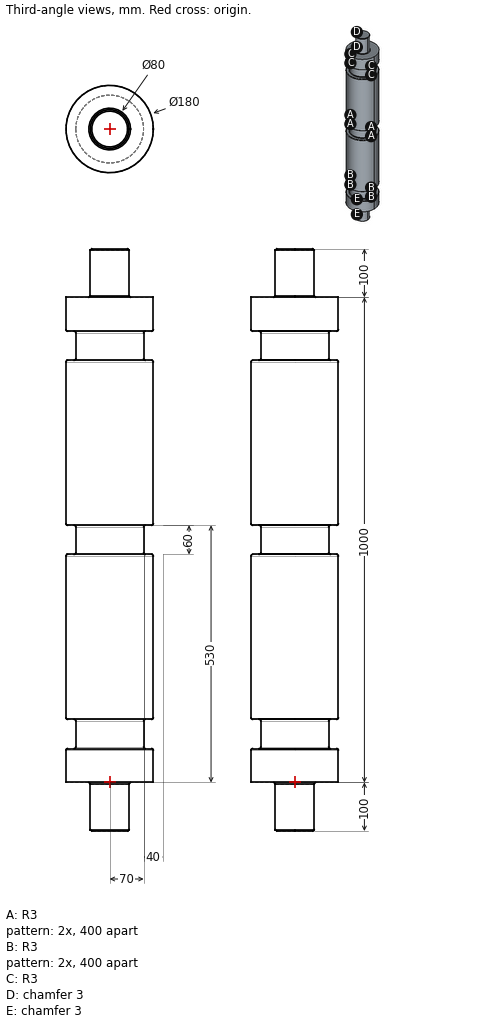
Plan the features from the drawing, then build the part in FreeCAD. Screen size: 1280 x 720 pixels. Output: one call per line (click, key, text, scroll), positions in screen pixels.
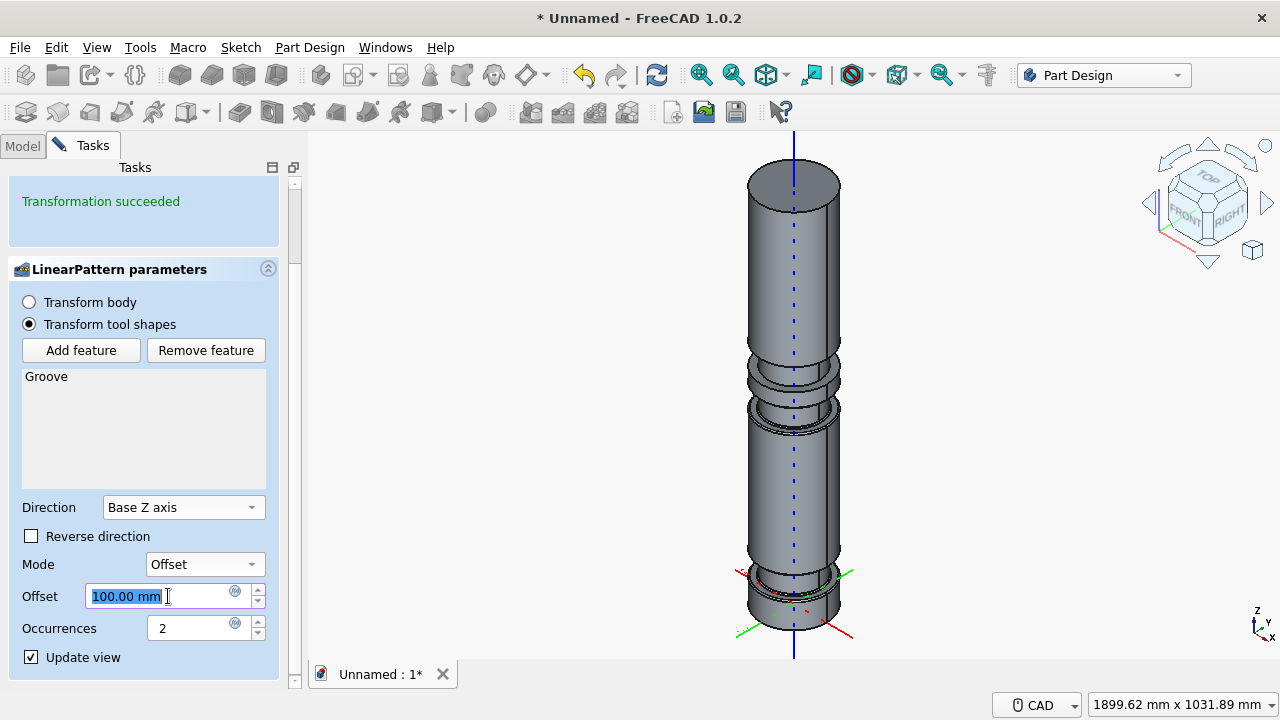
text(400)
key(Tab)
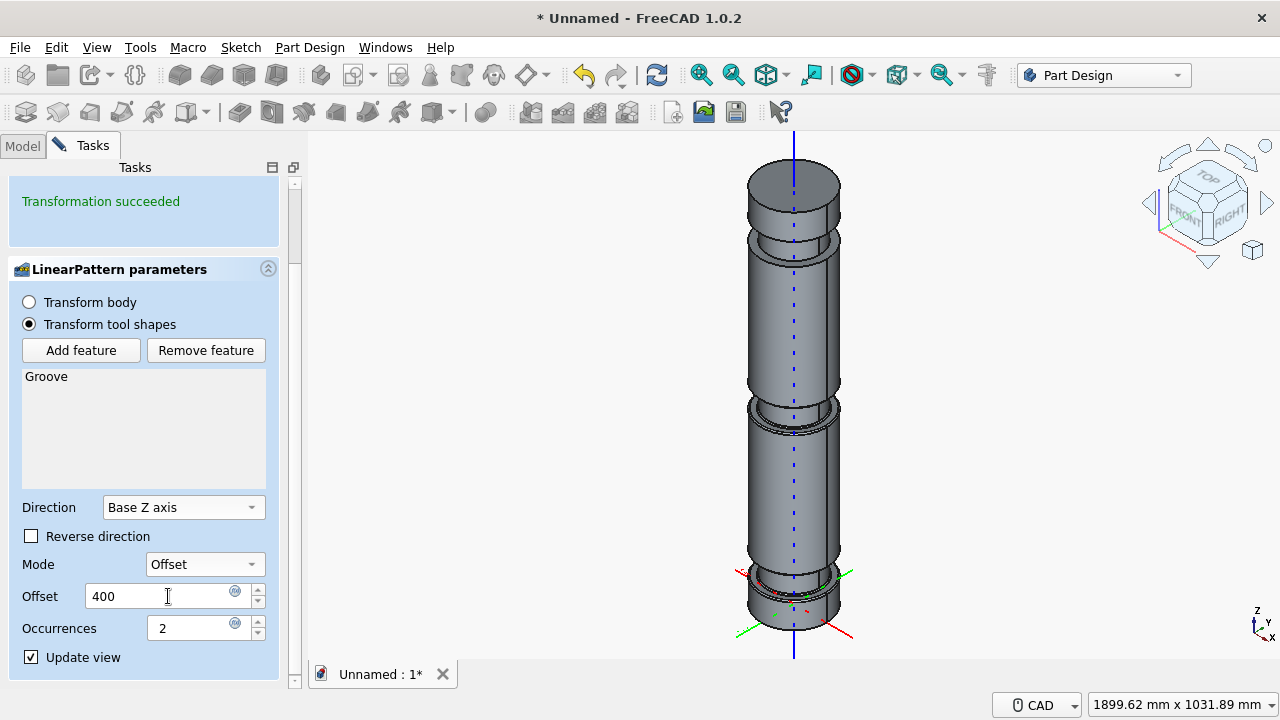
triple_click(198, 628)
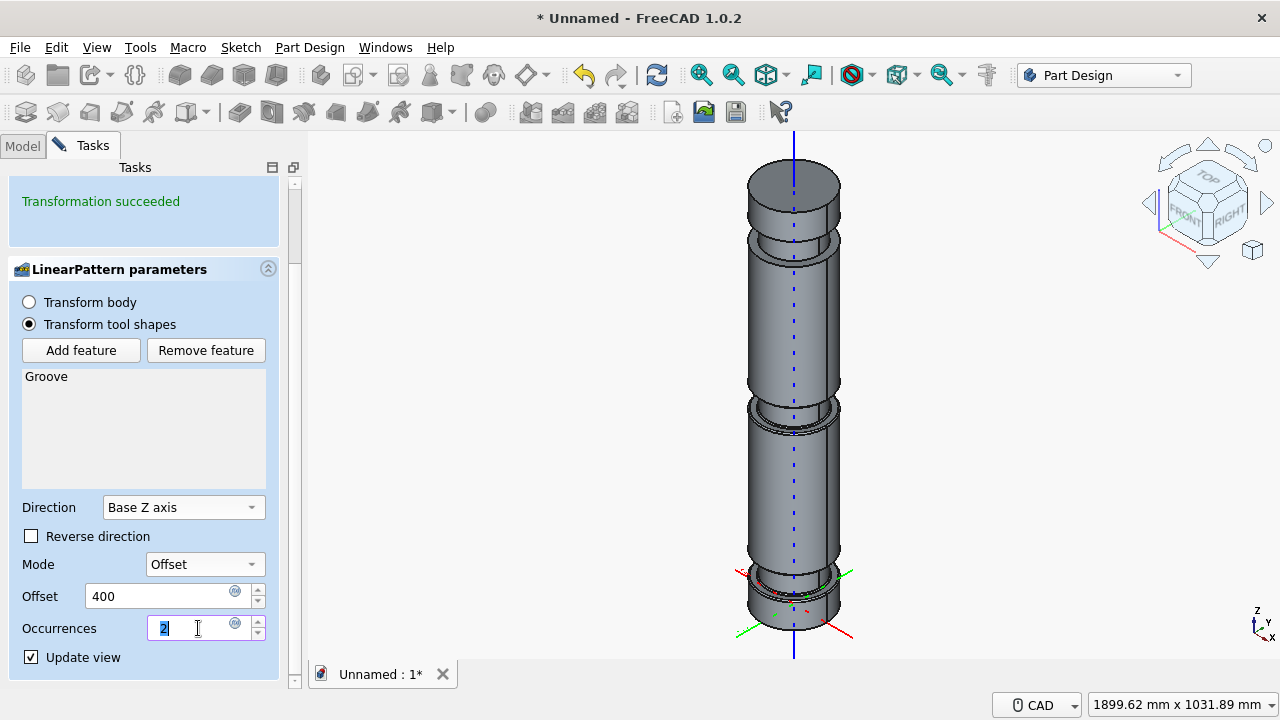
text(2)
key(Tab)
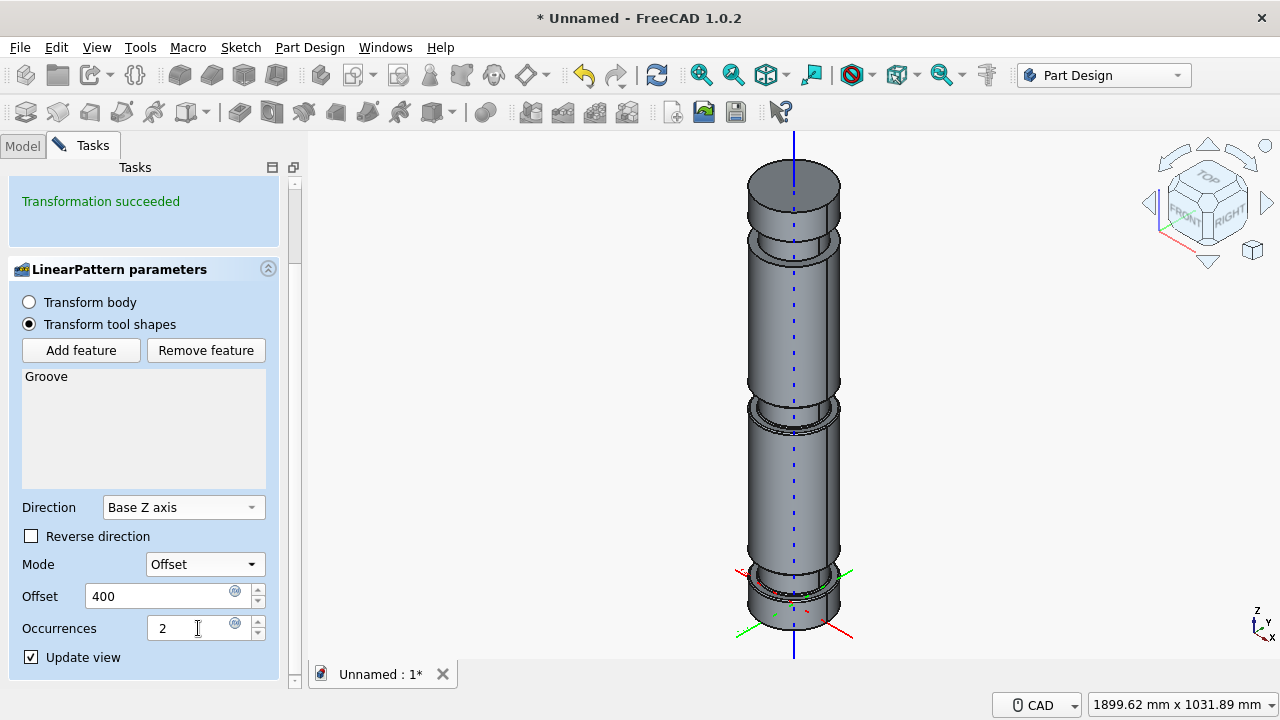
scroll(295, 432, up, 3)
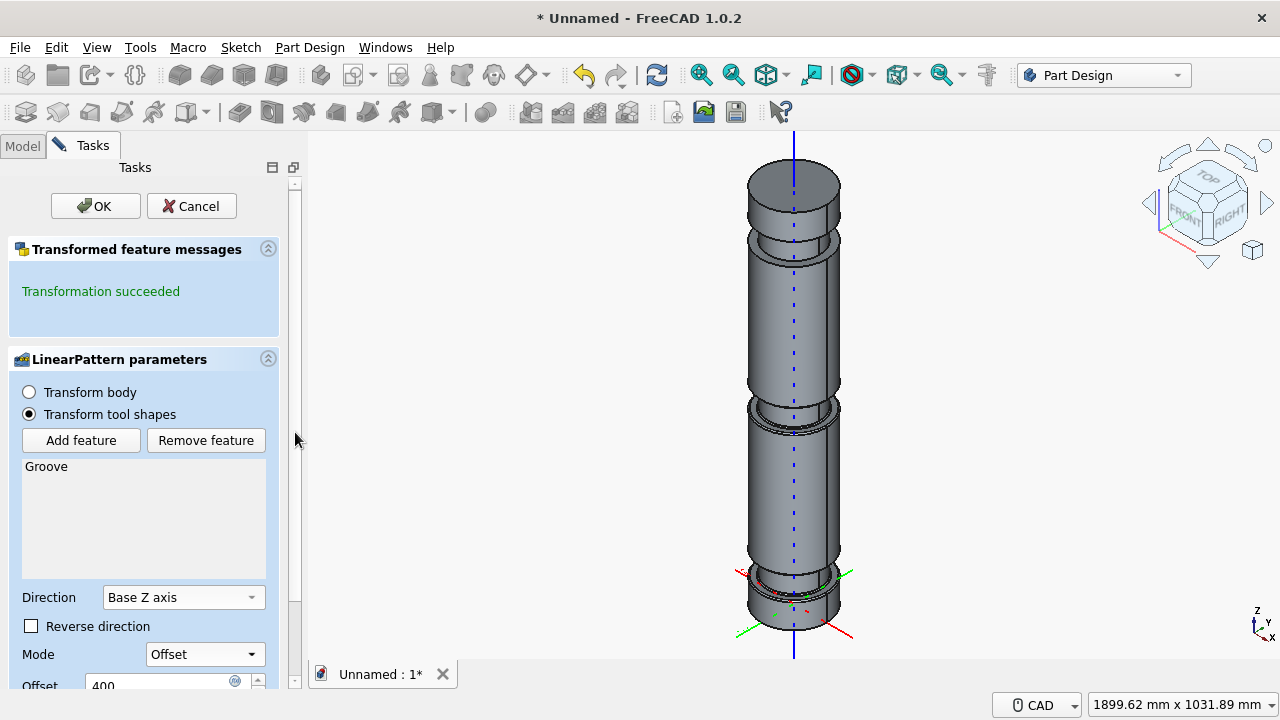
click(96, 206)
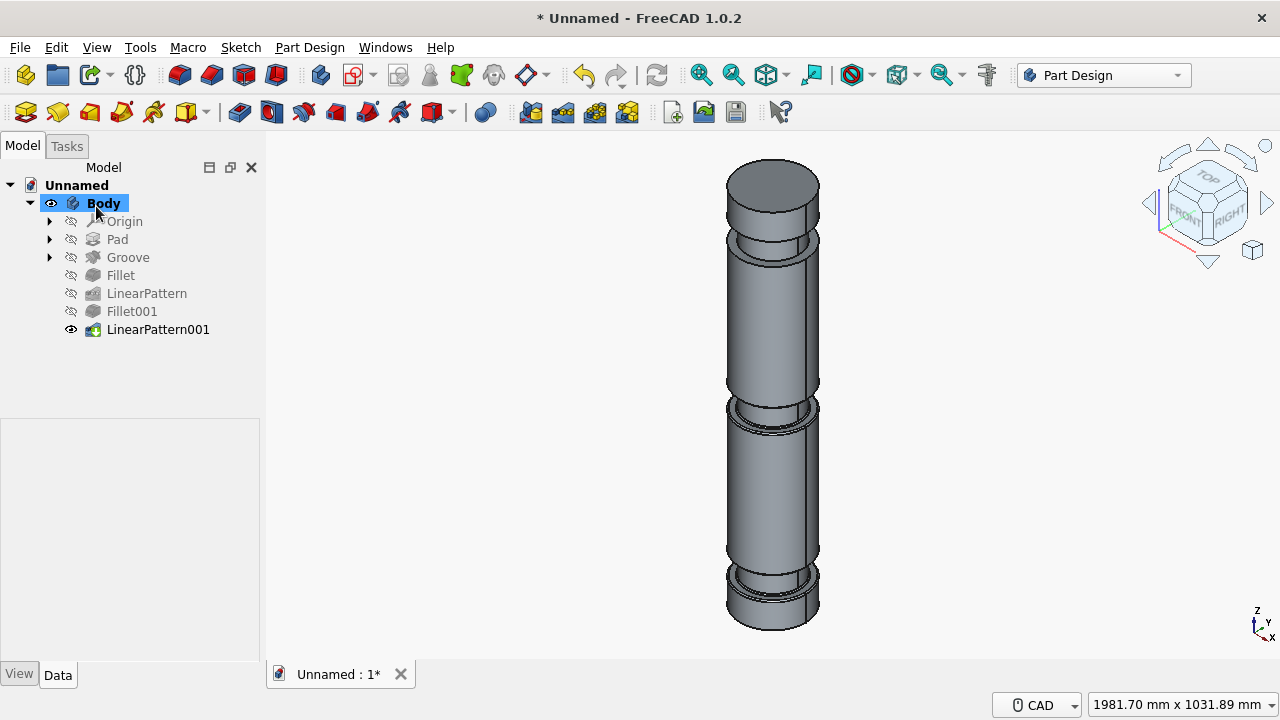
click(752, 238)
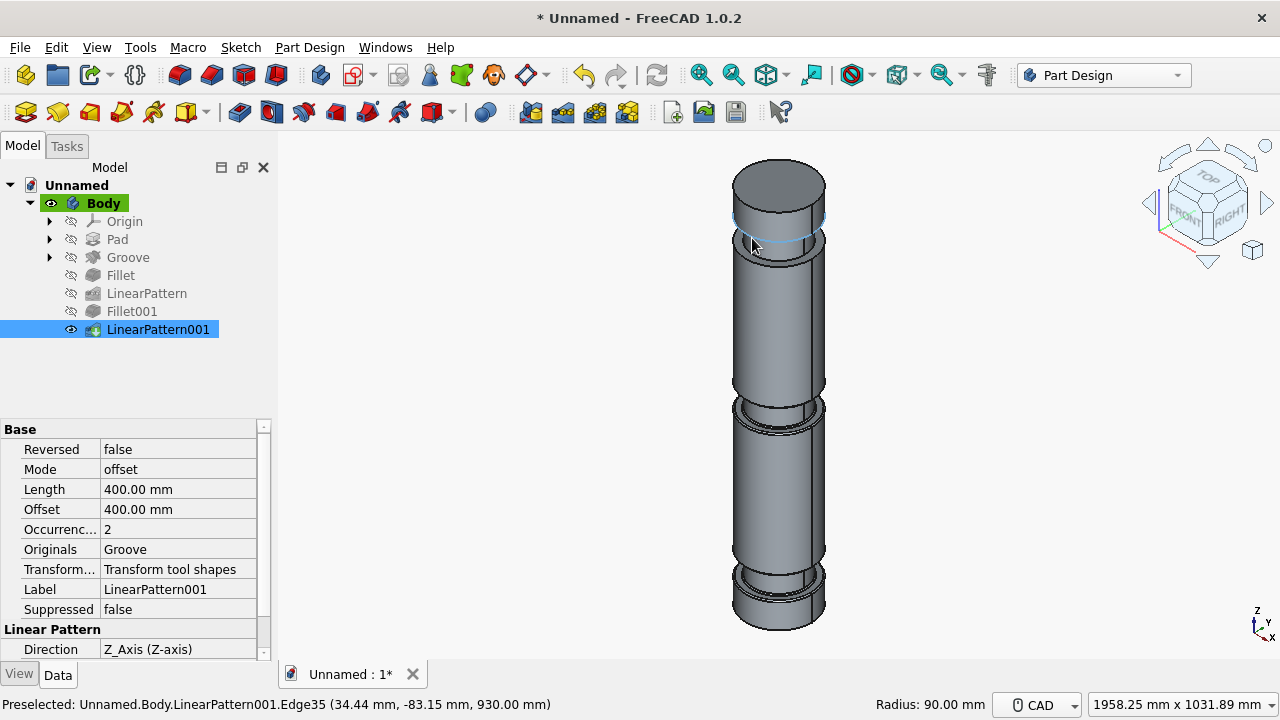
click(738, 251, ctrl)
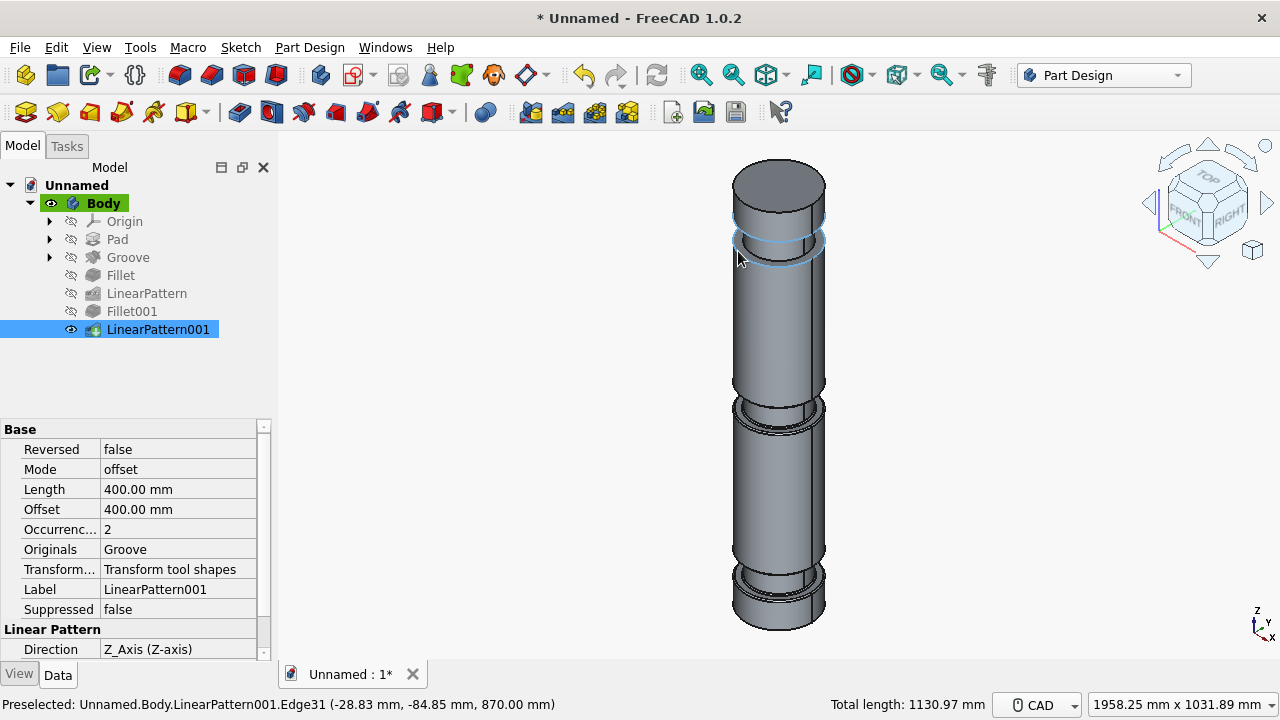
key(2)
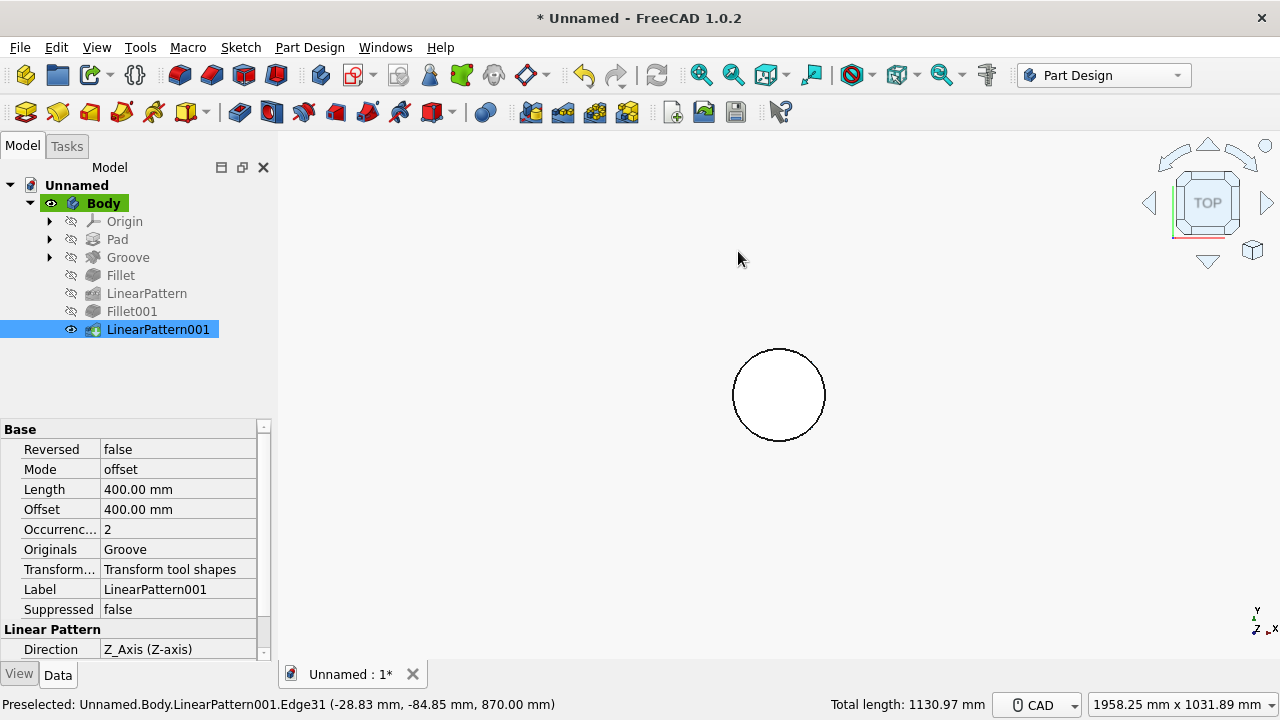
click(702, 76)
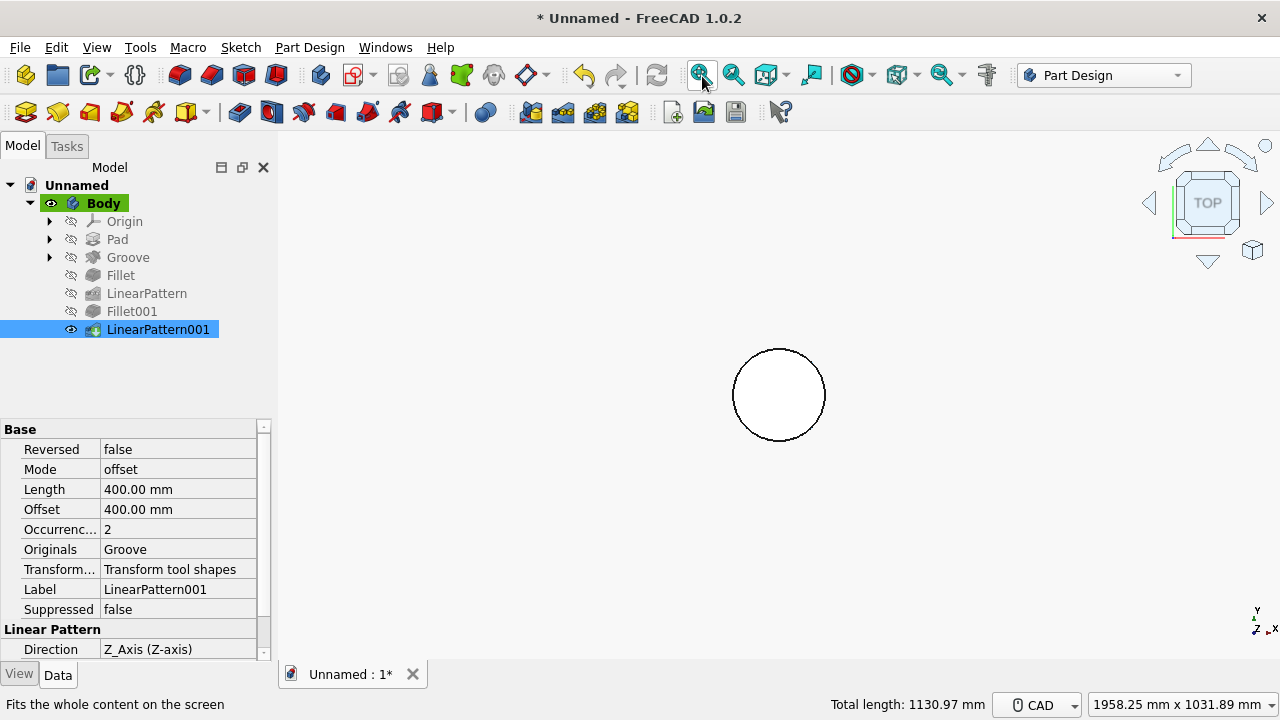
key(0)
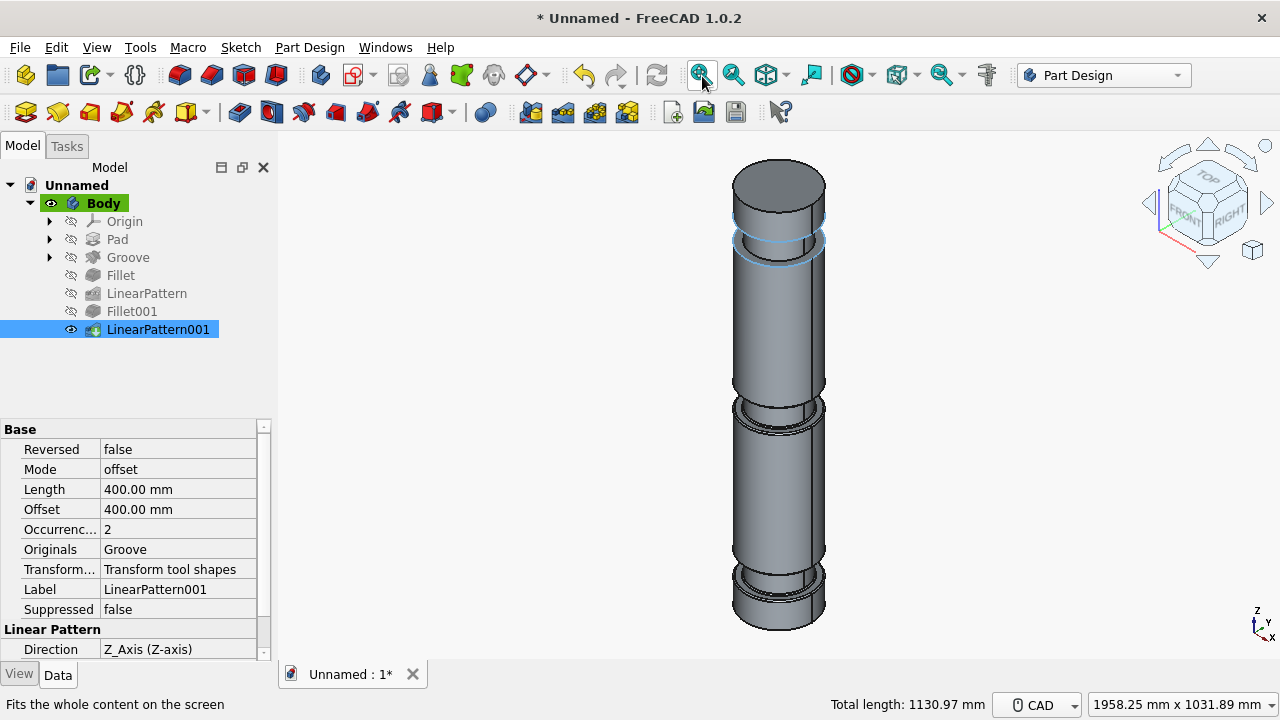
key(1)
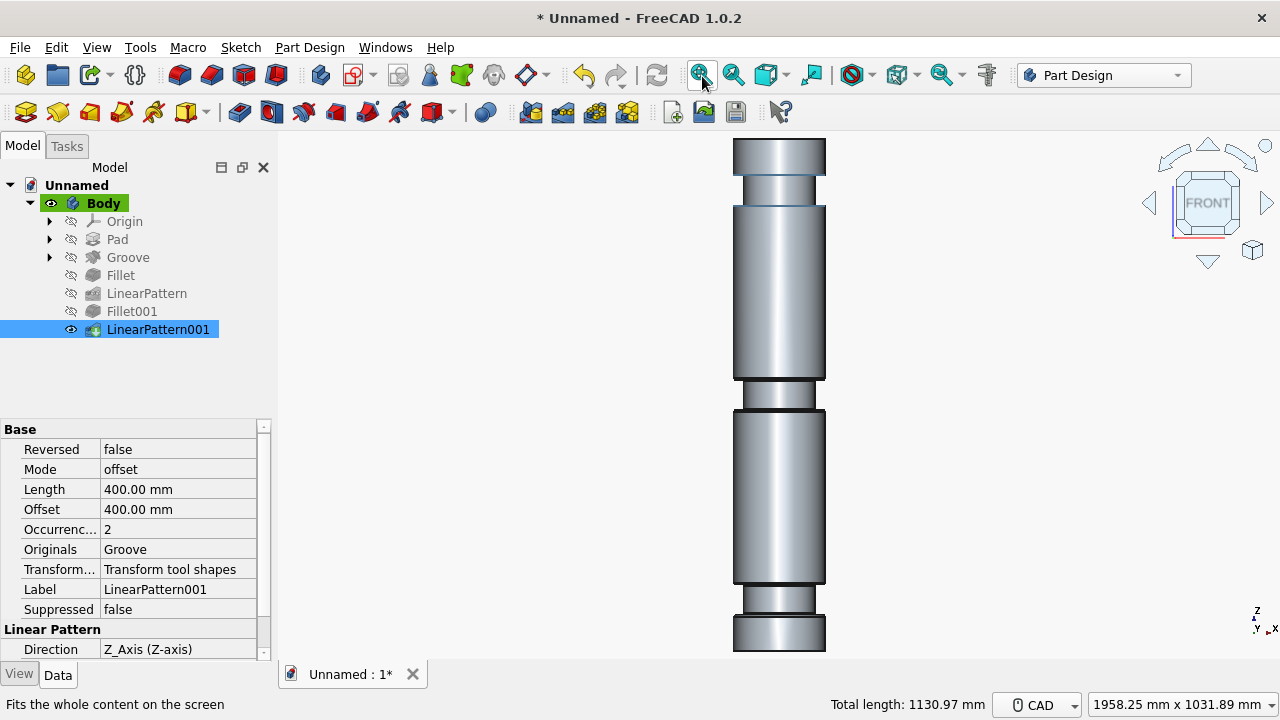
key(3)